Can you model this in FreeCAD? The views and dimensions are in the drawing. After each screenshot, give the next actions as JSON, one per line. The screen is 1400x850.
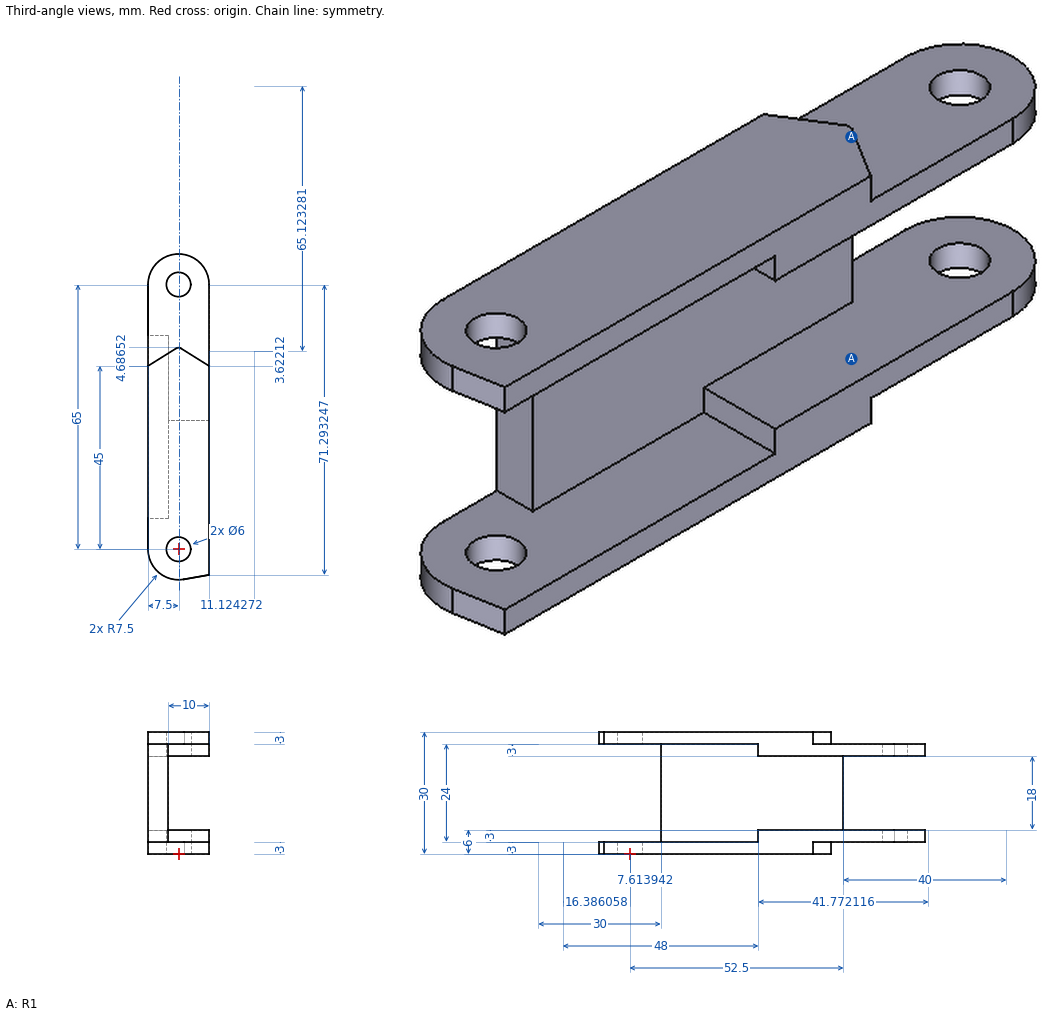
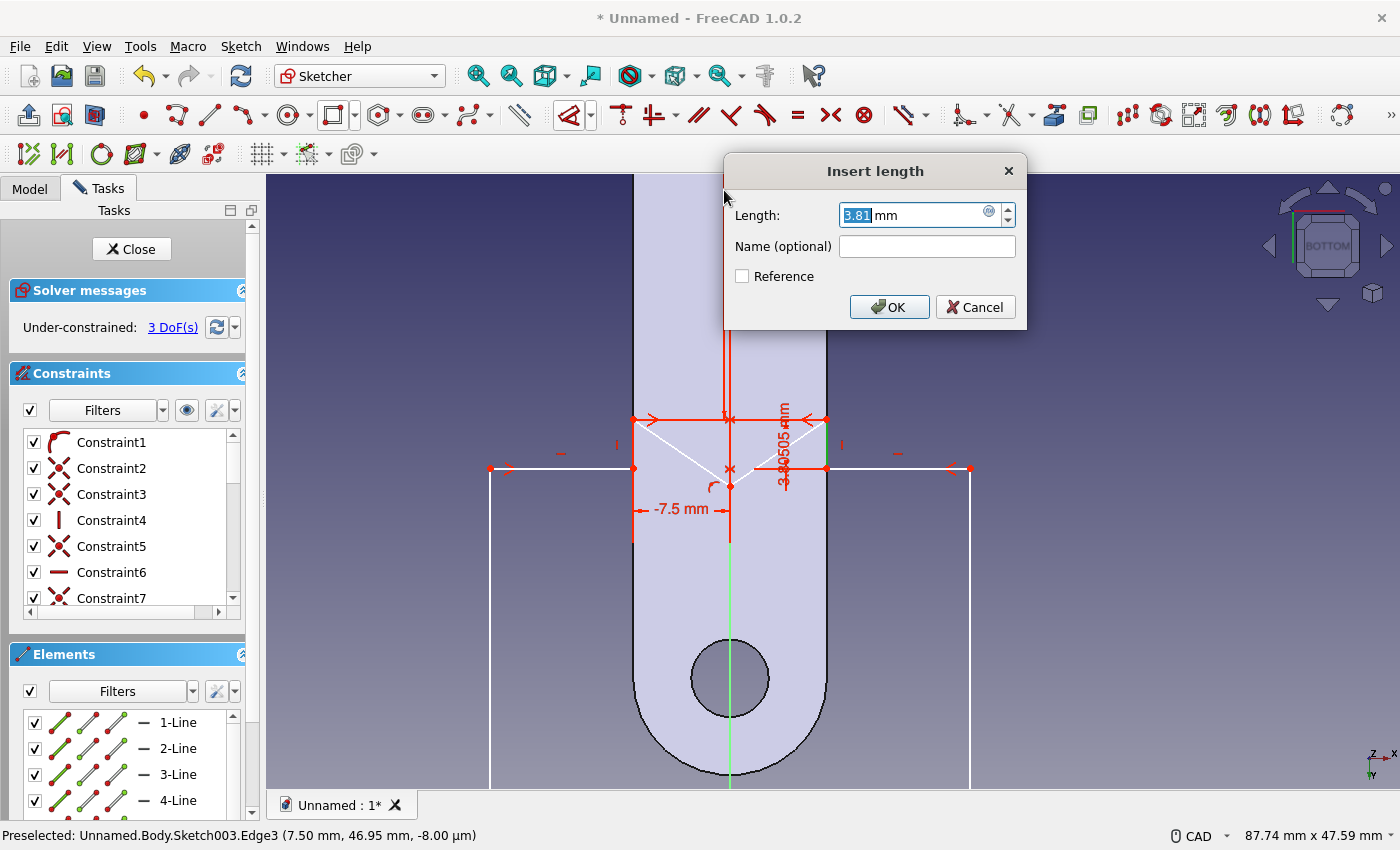
{"action": "type", "text": "3.62212"}
{"action": "key", "text": "Return"}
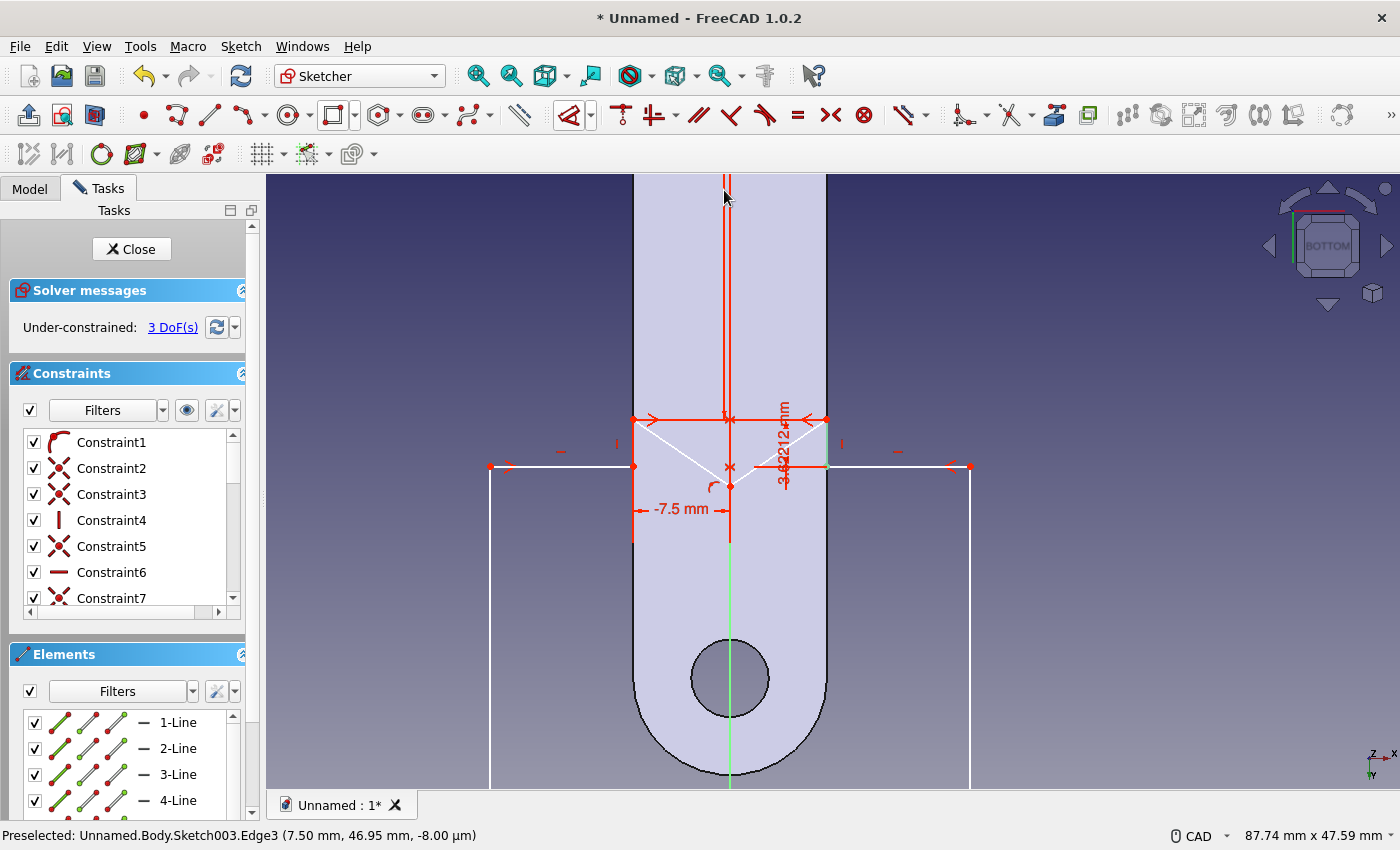
{"action": "left_click", "coordinate": [662, 440]}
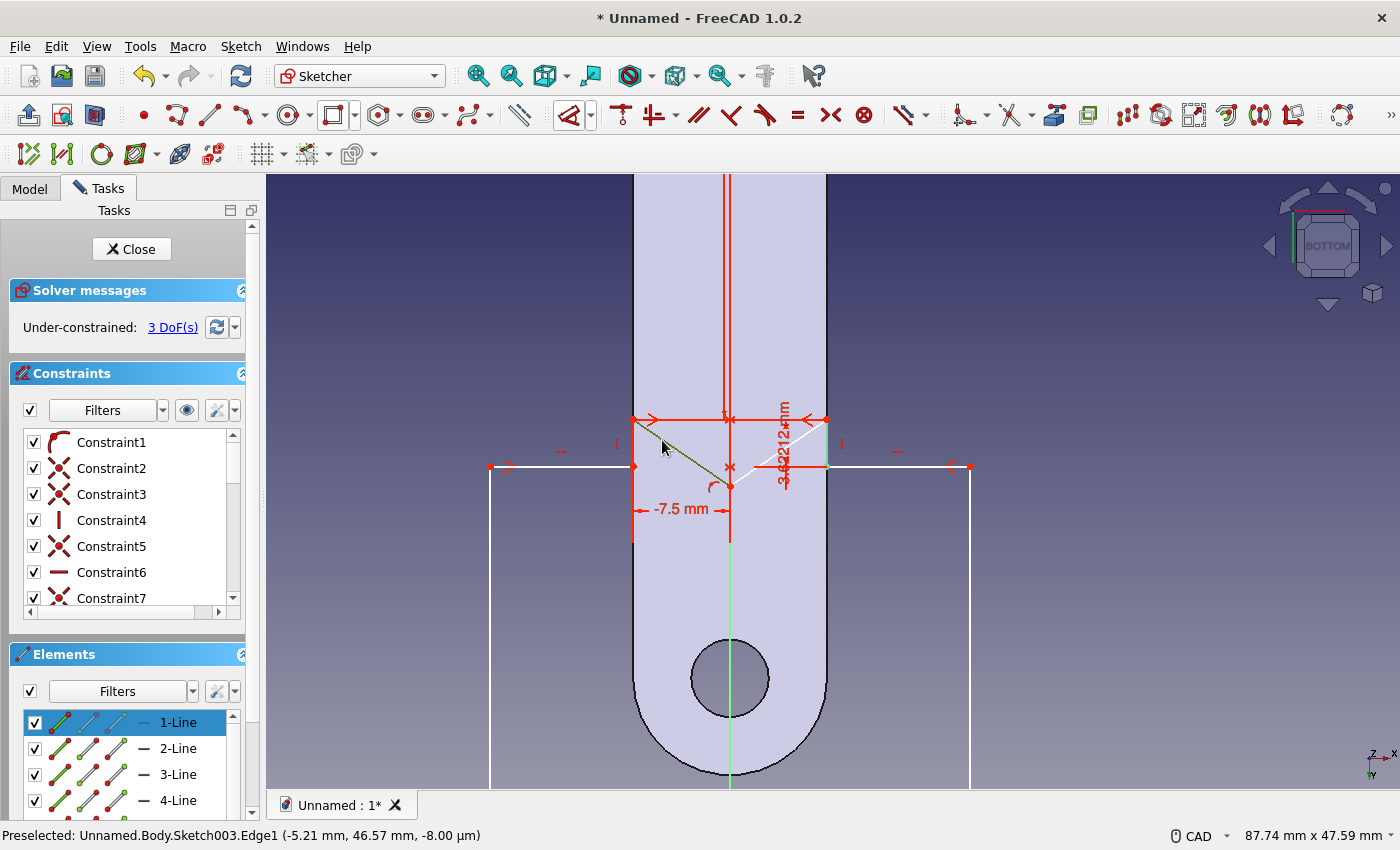
{"action": "key", "text": "i"}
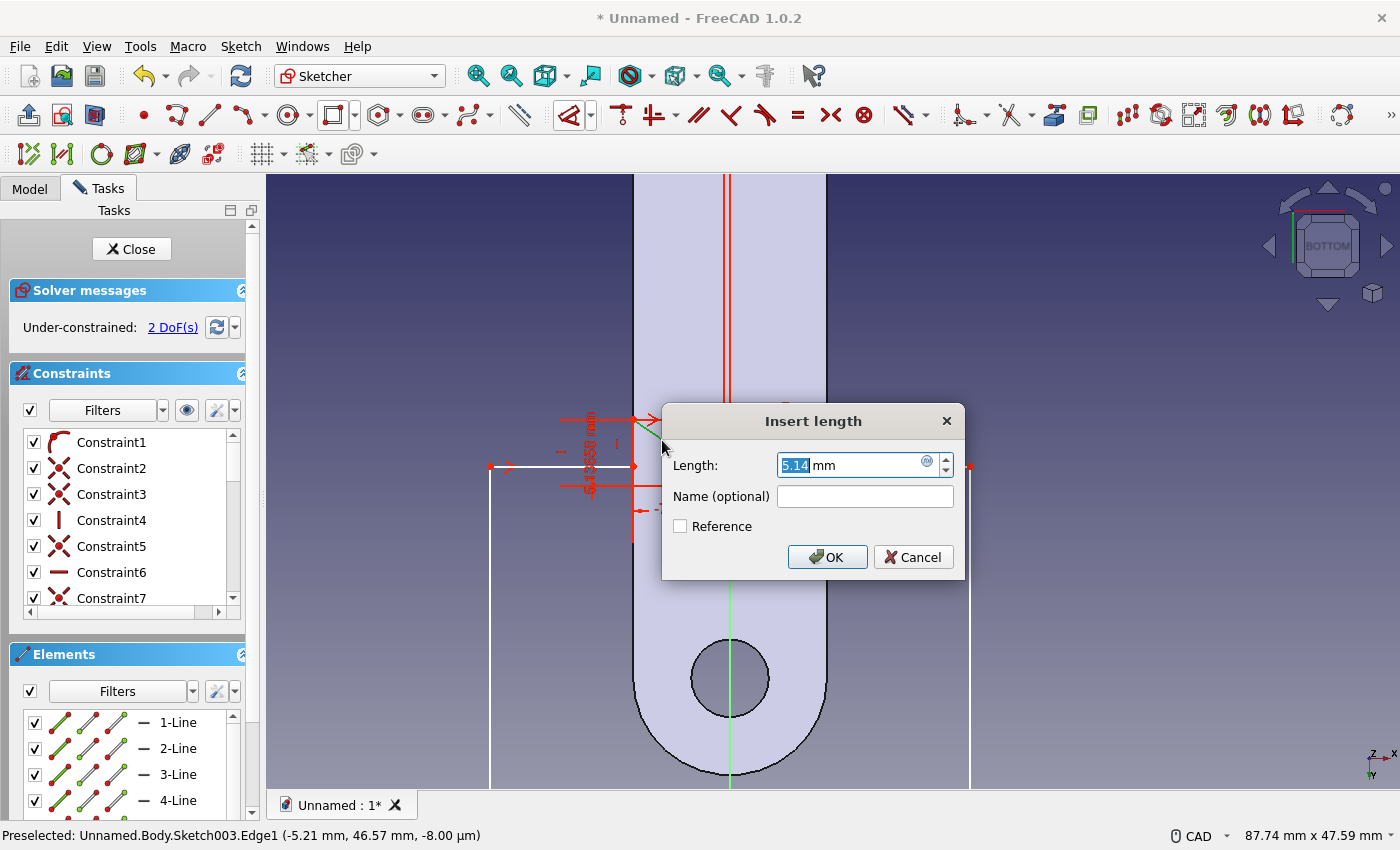
{"action": "type", "text": "4.68652"}
{"action": "key", "text": "Return"}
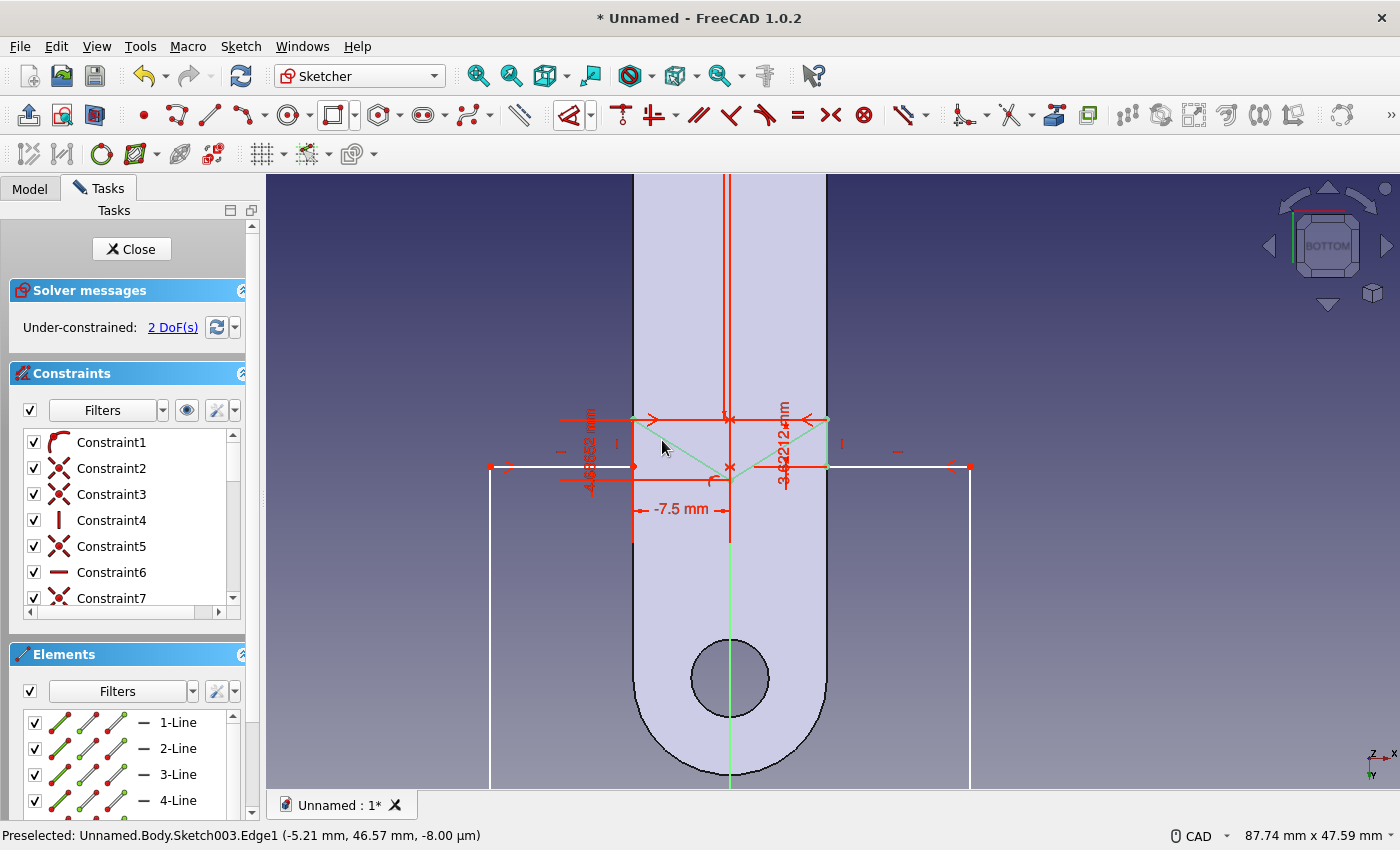
{"action": "scroll", "coordinate": [776, 451], "scroll_direction": "down", "scroll_amount": 7}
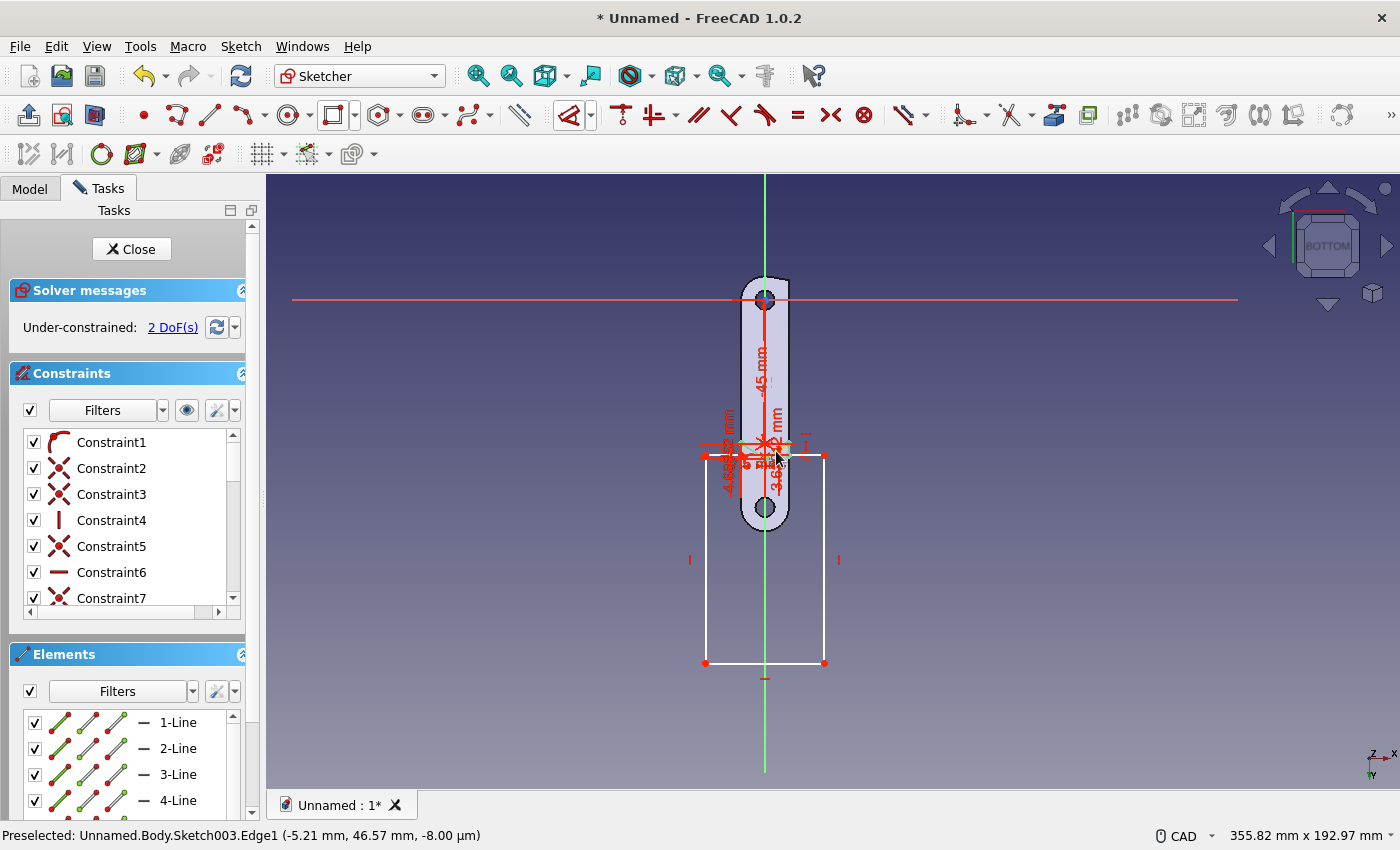
{"action": "scroll", "coordinate": [799, 455], "scroll_direction": "up", "scroll_amount": 2}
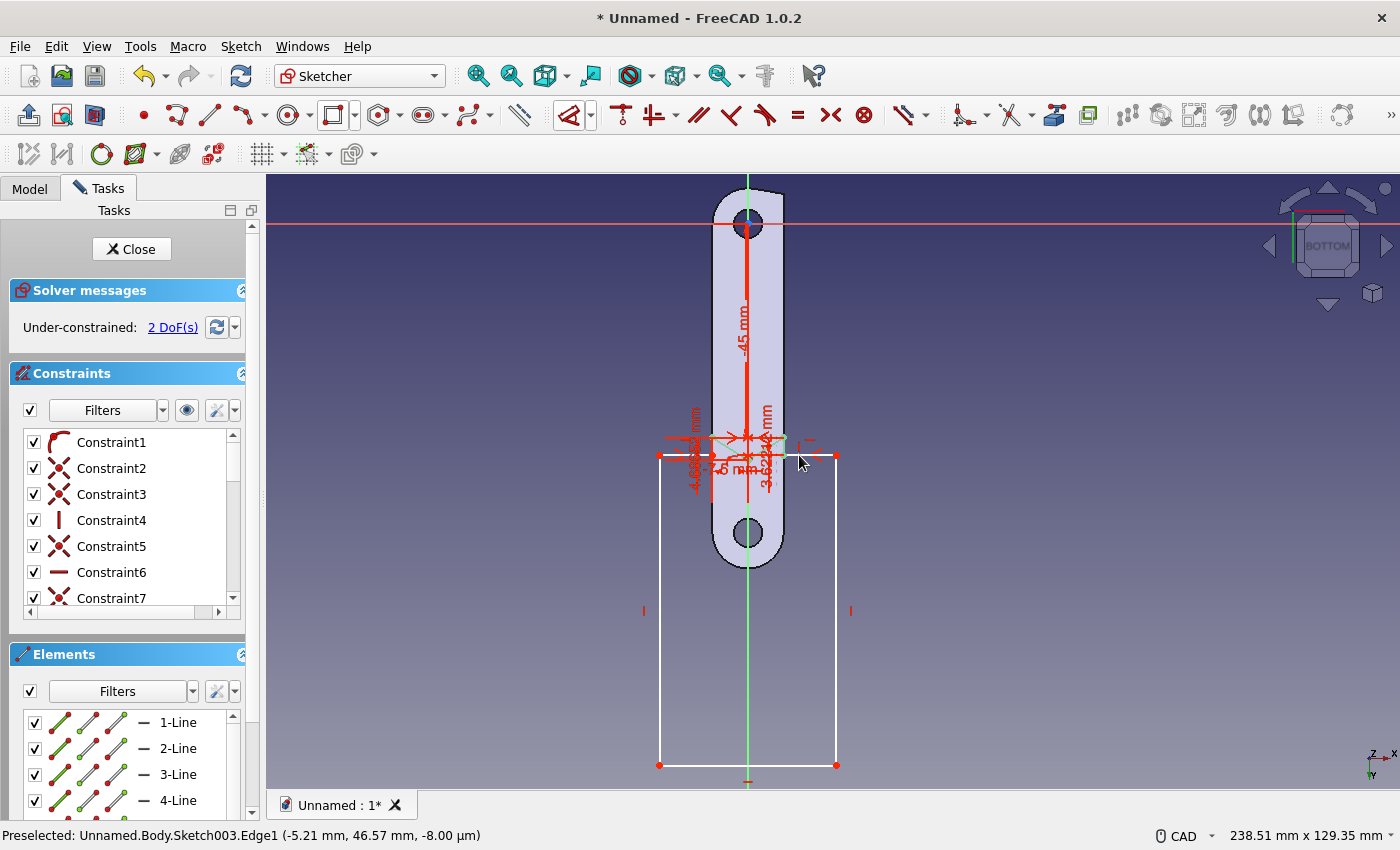
{"action": "left_click", "coordinate": [800, 455]}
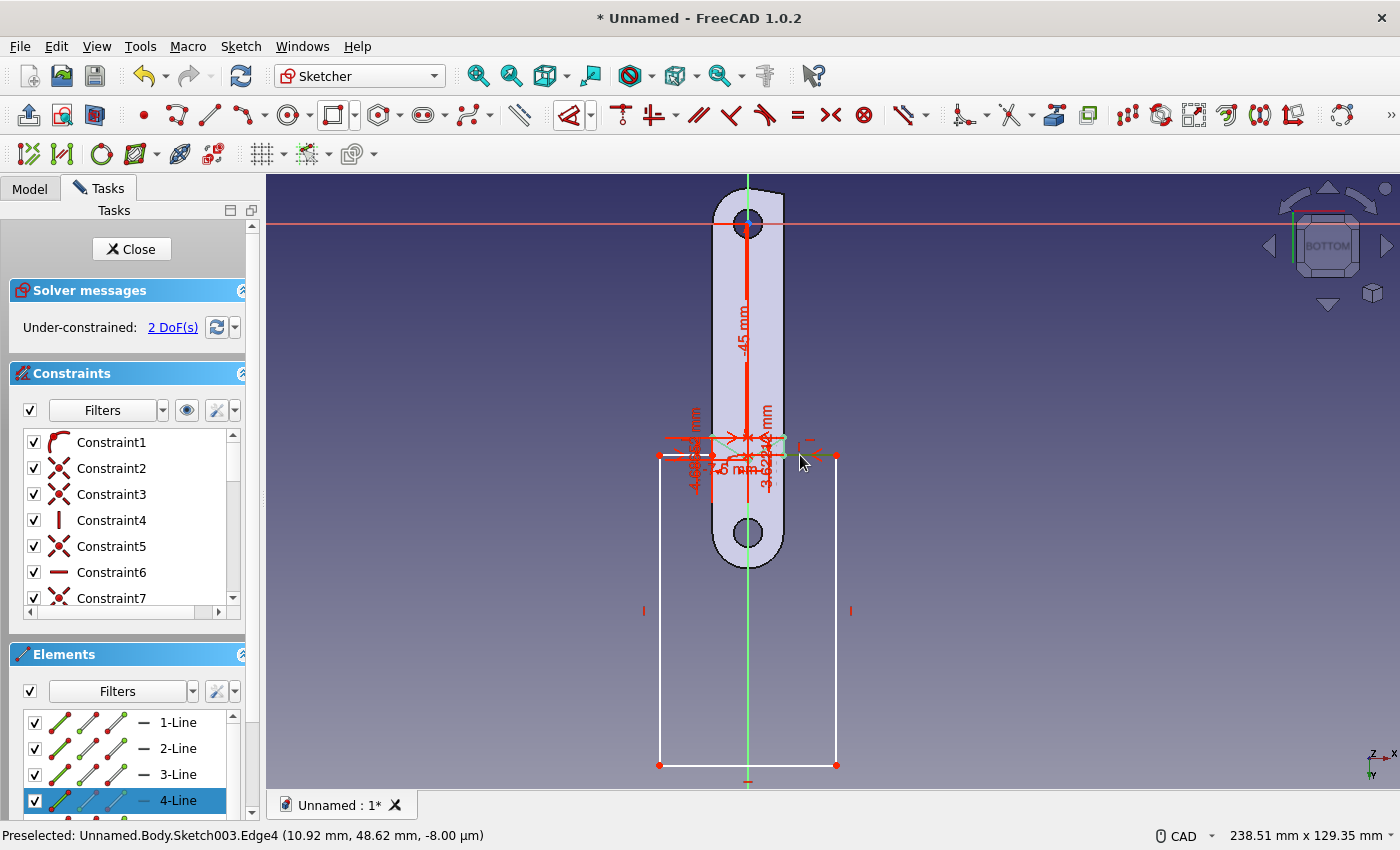
{"action": "key", "text": "l"}